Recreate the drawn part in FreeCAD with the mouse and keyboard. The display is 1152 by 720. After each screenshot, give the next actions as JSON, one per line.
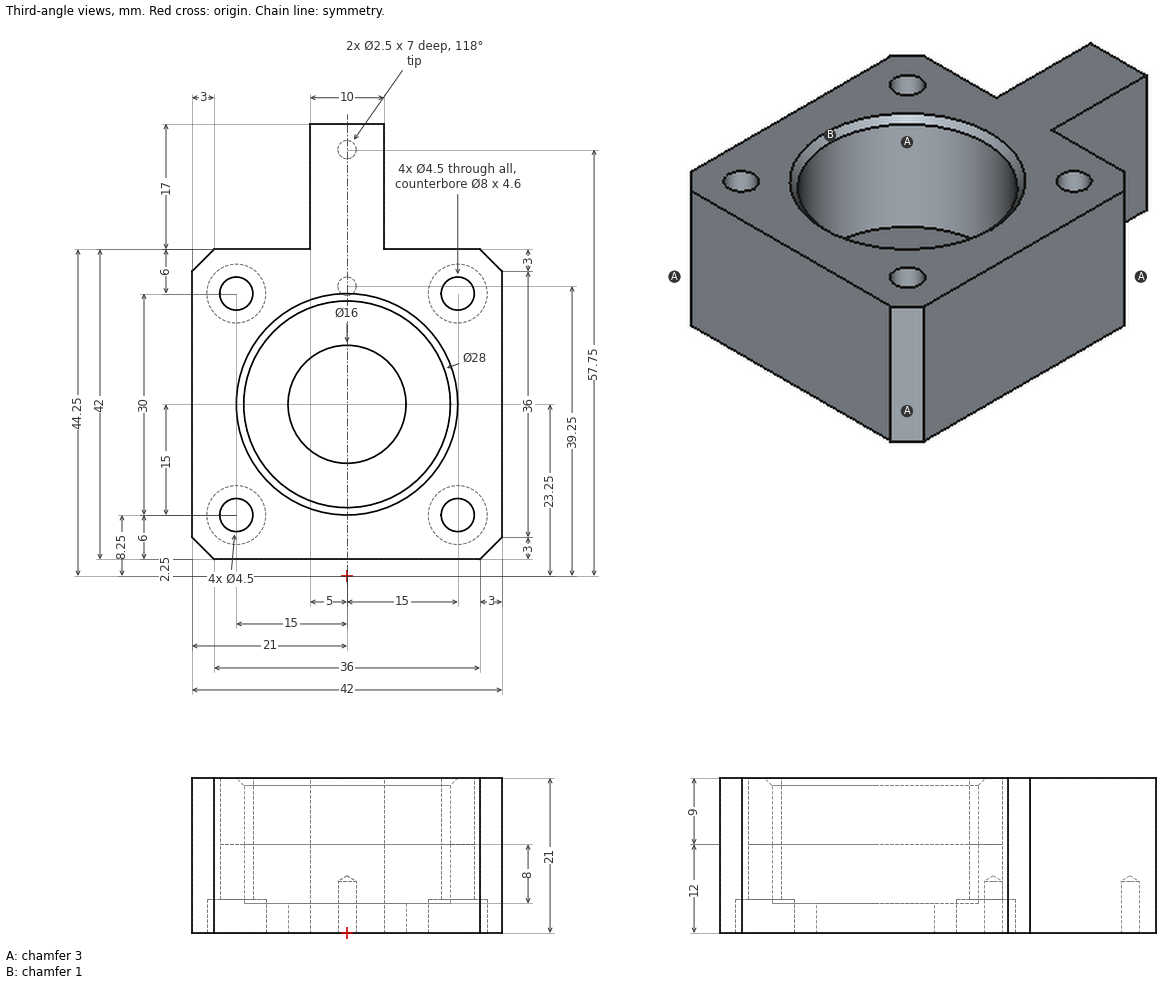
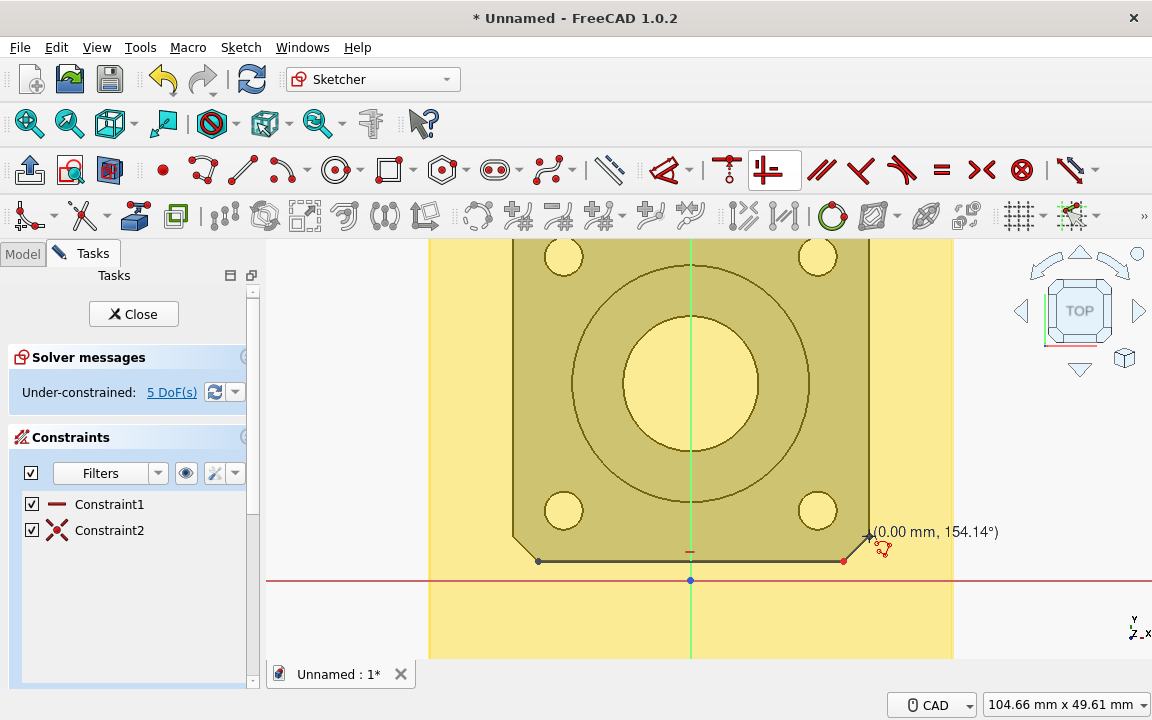
{"action": "scroll", "coordinate": [538, 562], "scroll_direction": "down", "scroll_amount": 2}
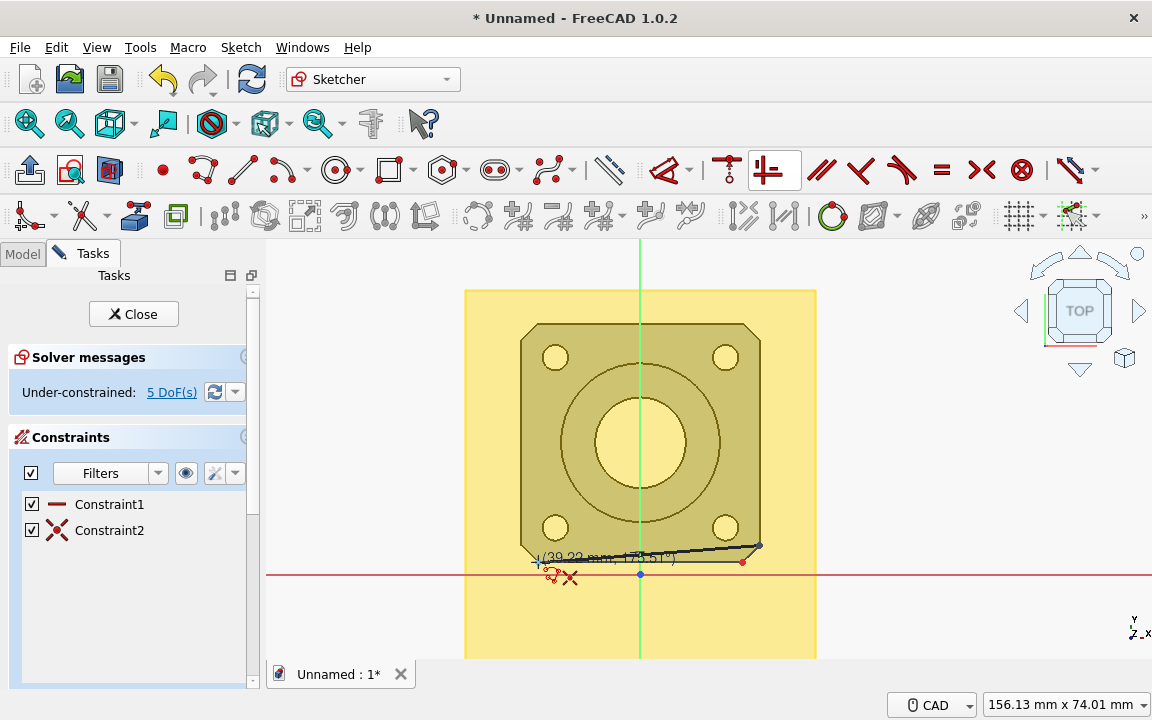
{"action": "left_click", "coordinate": [760, 341]}
{"action": "left_click", "coordinate": [743, 324]}
{"action": "left_click", "coordinate": [538, 324]}
{"action": "left_click", "coordinate": [521, 341]}
{"action": "left_click", "coordinate": [521, 545]}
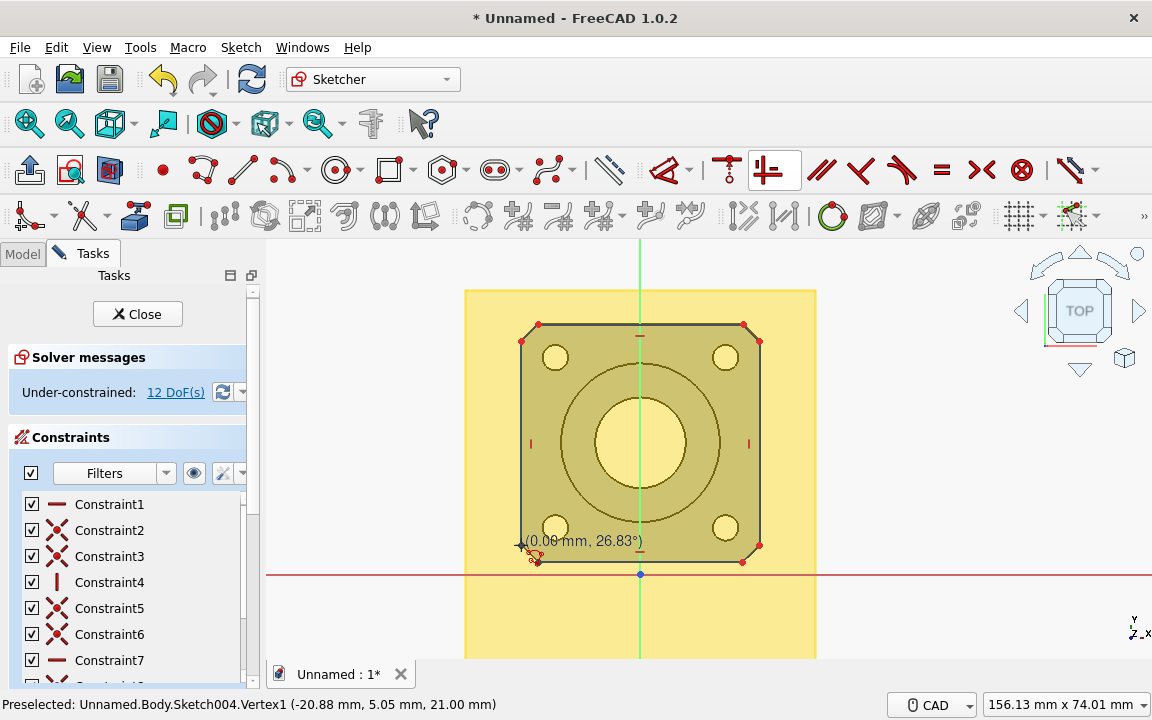
{"action": "scroll", "coordinate": [538, 562], "scroll_direction": "up", "scroll_amount": 2}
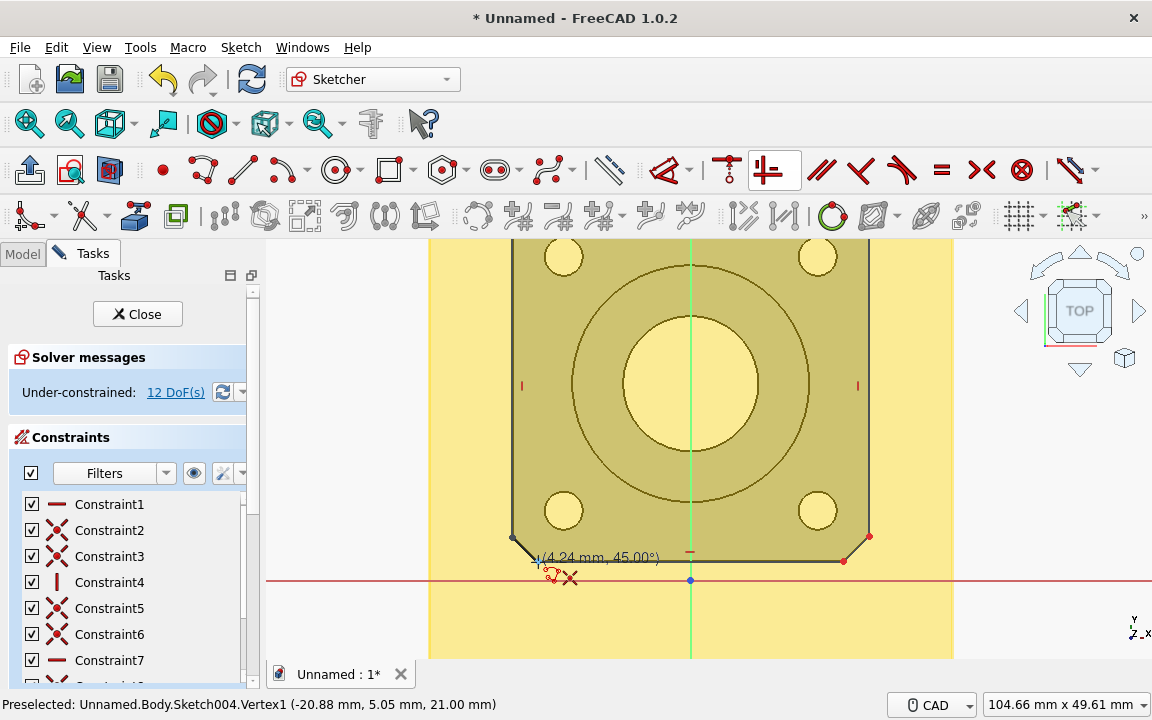
{"action": "left_click", "coordinate": [538, 562]}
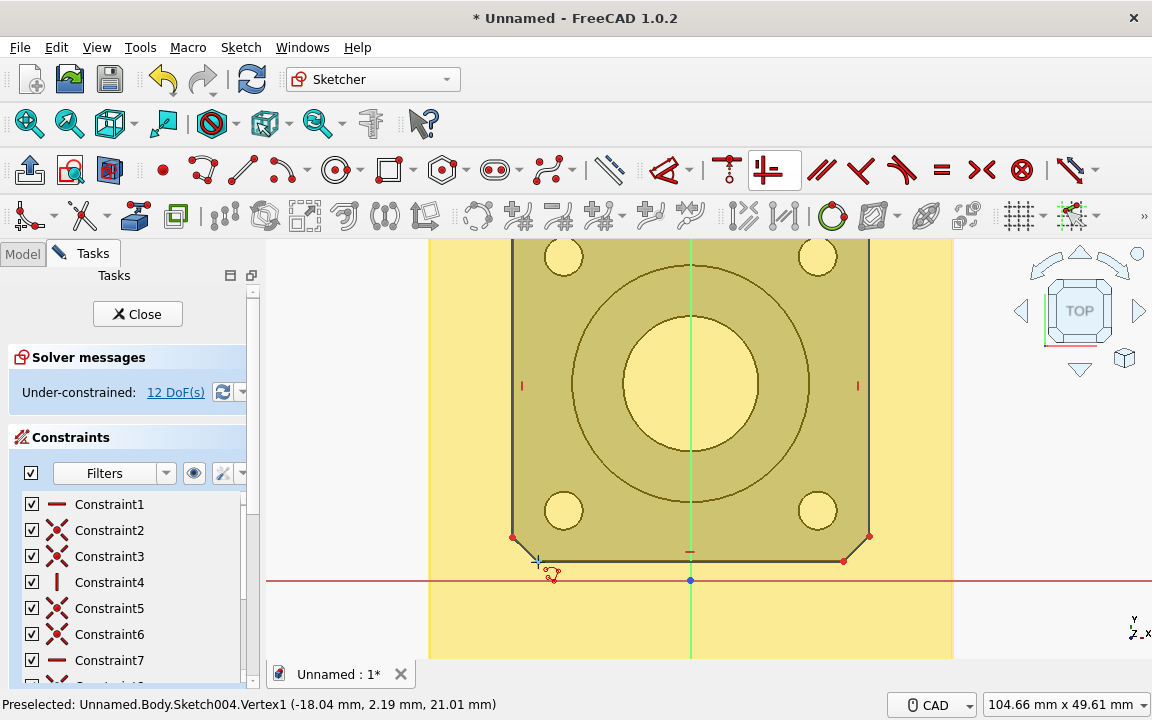
{"action": "left_click", "coordinate": [336, 170]}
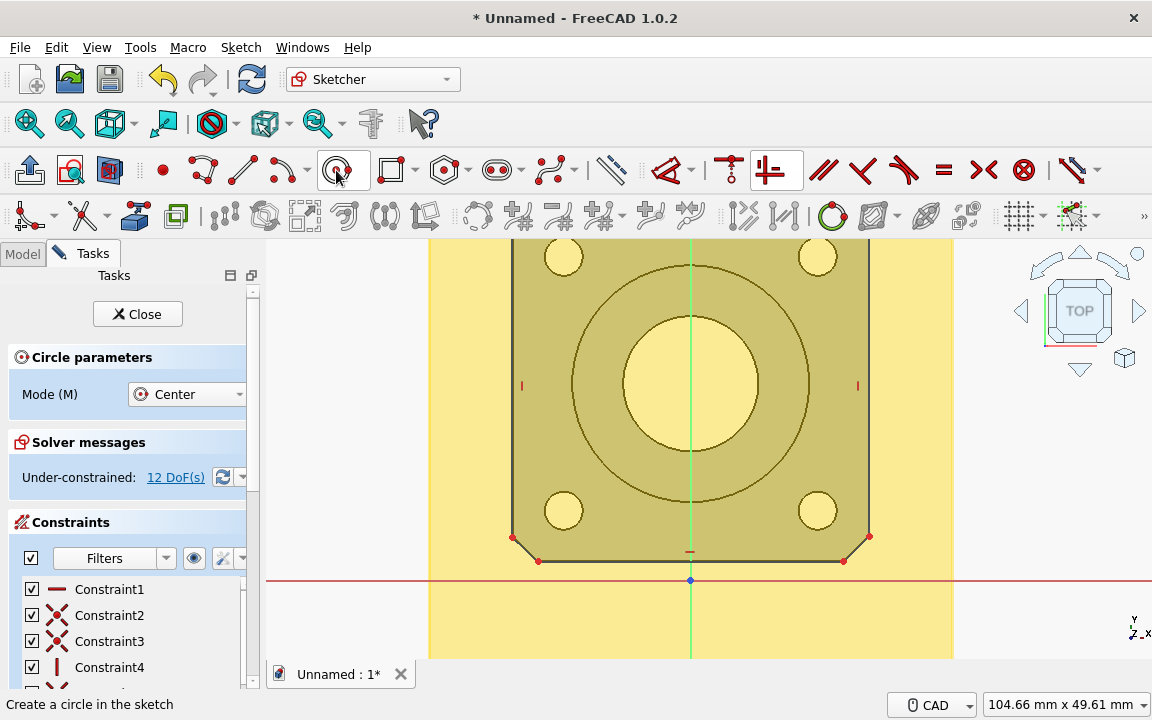
{"action": "left_click", "coordinate": [564, 511]}
{"action": "left_click", "coordinate": [577, 497]}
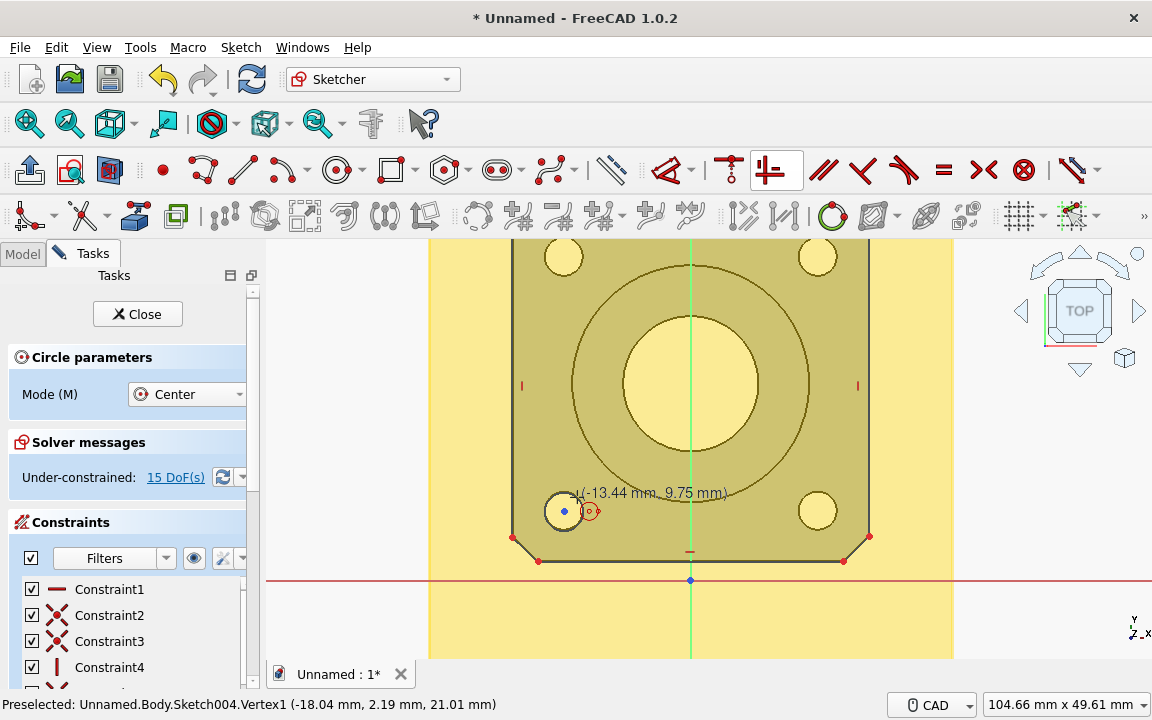
{"action": "left_click", "coordinate": [818, 511]}
{"action": "left_click", "coordinate": [831, 497]}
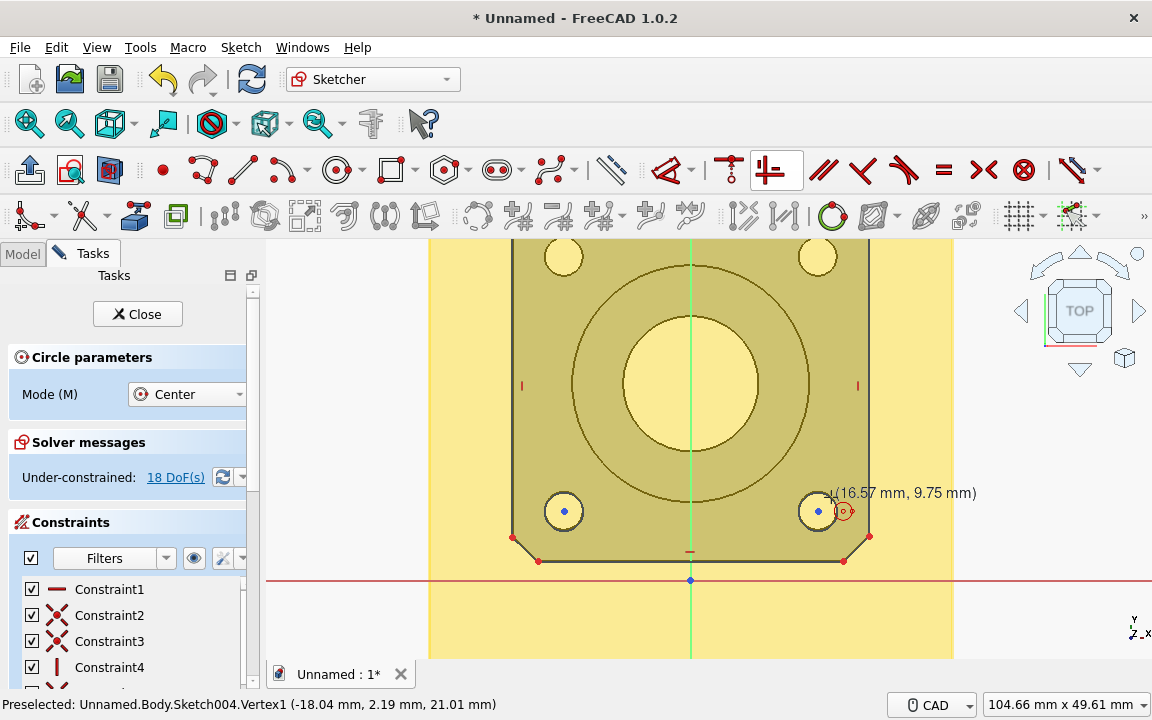
{"action": "scroll", "coordinate": [538, 562], "scroll_direction": "down", "scroll_amount": 2}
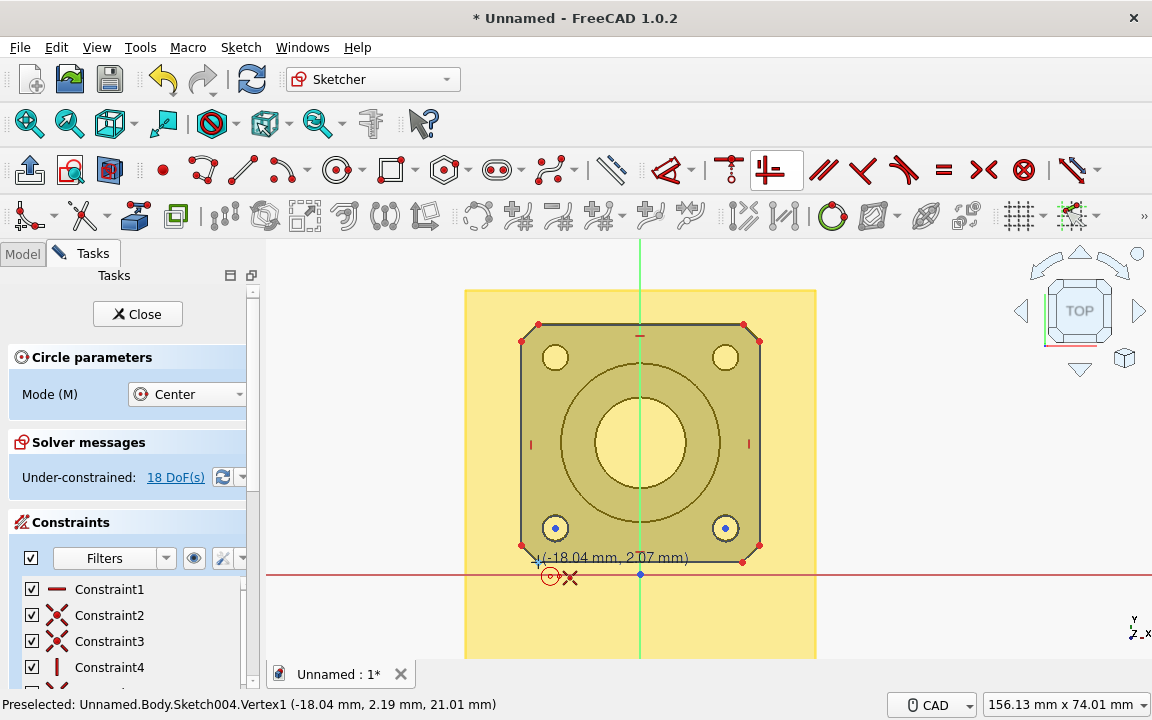
{"action": "scroll", "coordinate": [555, 358], "scroll_direction": "up", "scroll_amount": 3}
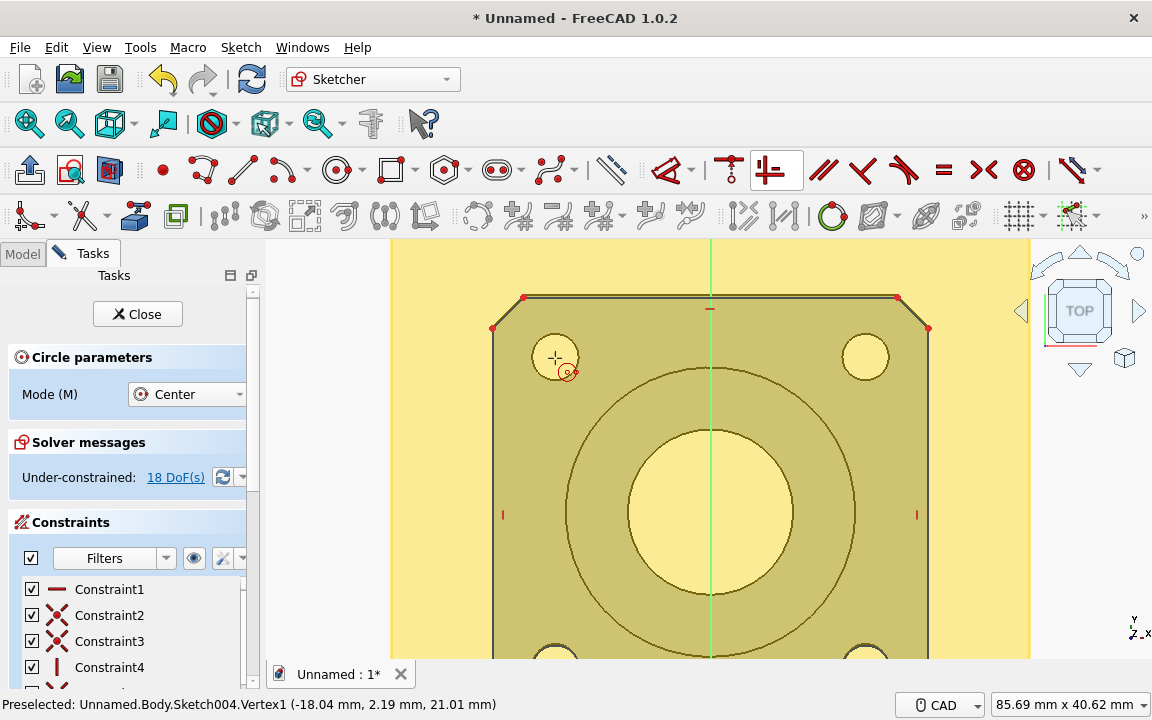
{"action": "left_click", "coordinate": [555, 357]}
{"action": "left_click", "coordinate": [572, 341]}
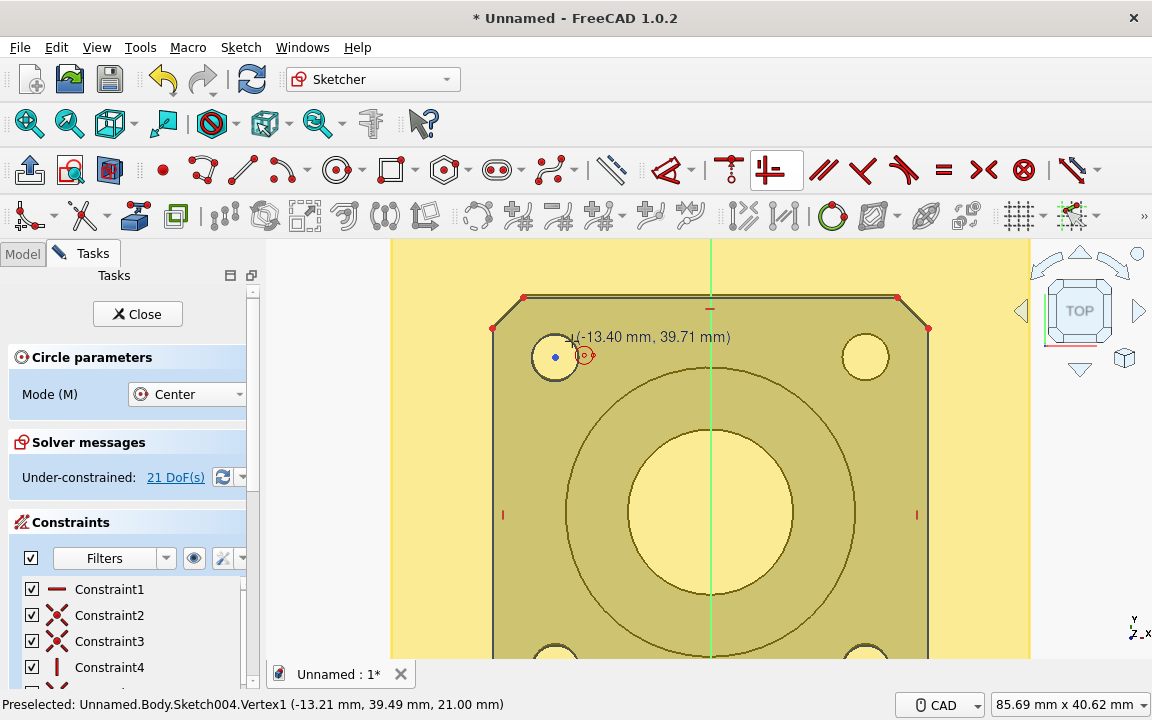
{"action": "left_click", "coordinate": [711, 512]}
{"action": "left_click", "coordinate": [813, 410]}